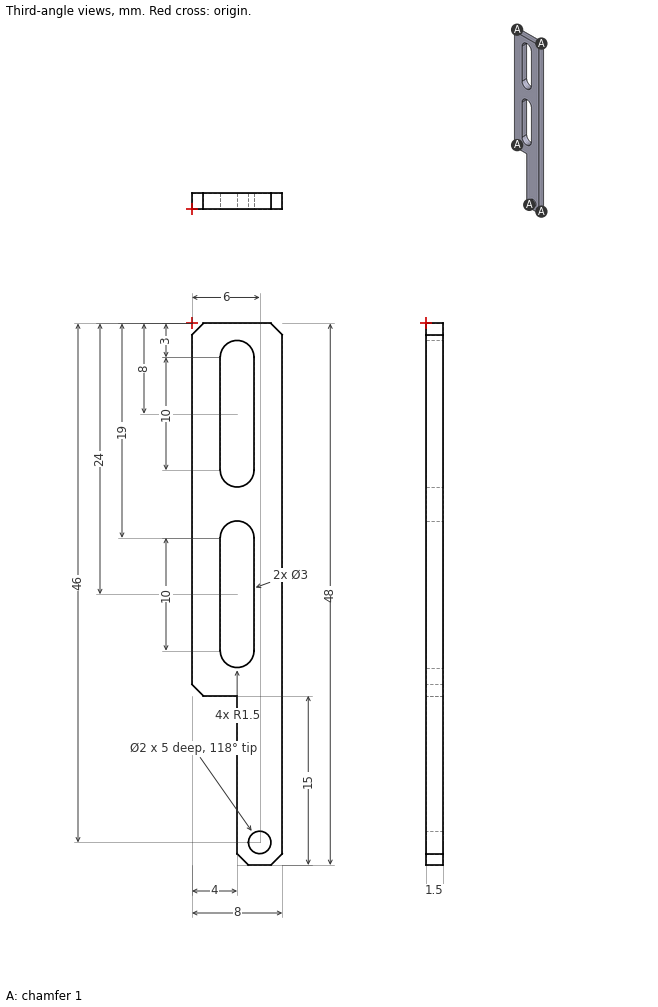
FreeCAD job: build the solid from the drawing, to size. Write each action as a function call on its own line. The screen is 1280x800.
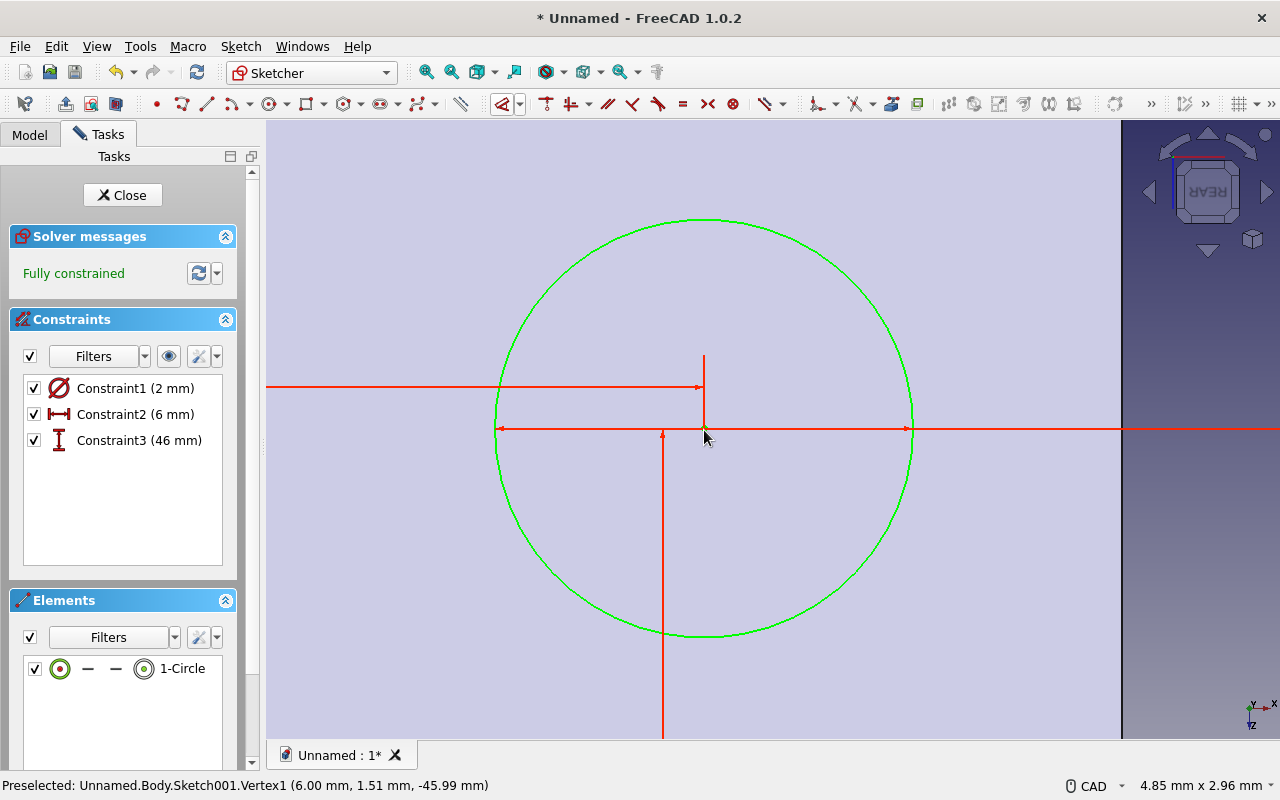
click(123, 195)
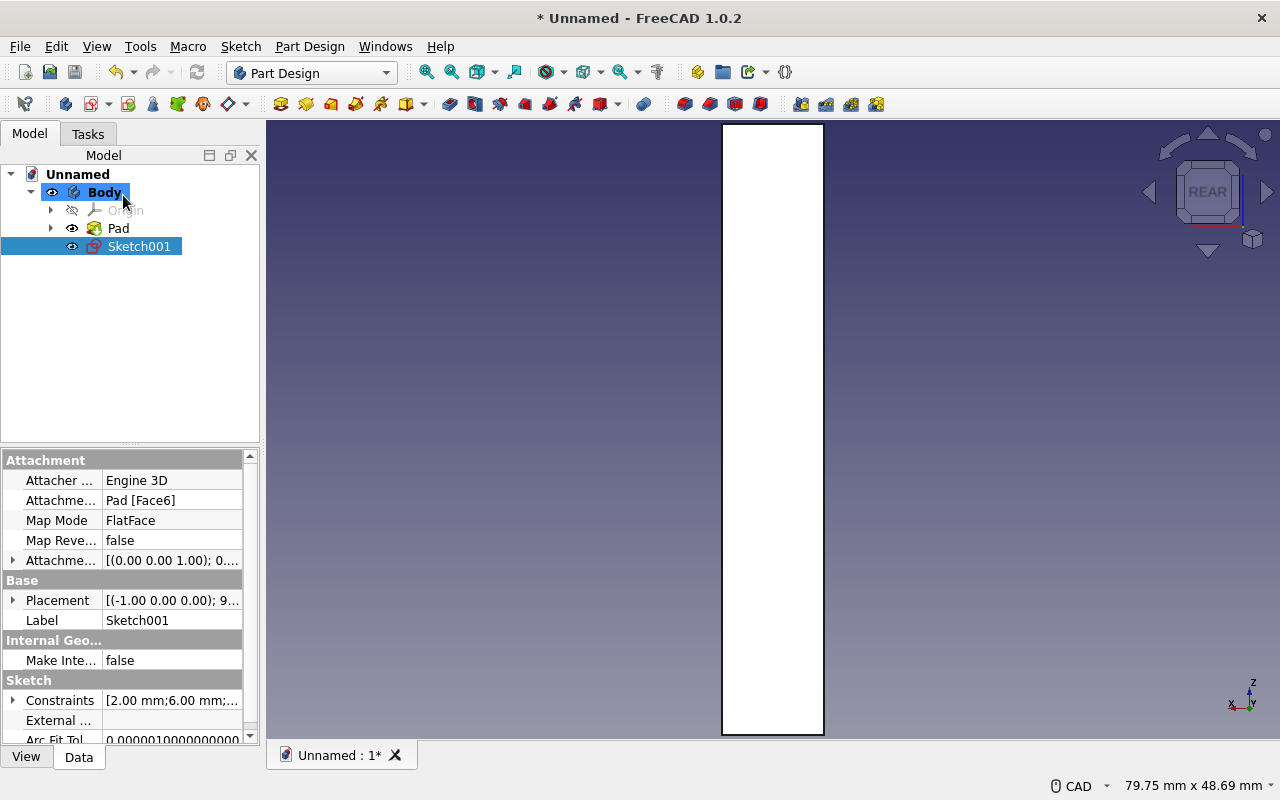
click(475, 104)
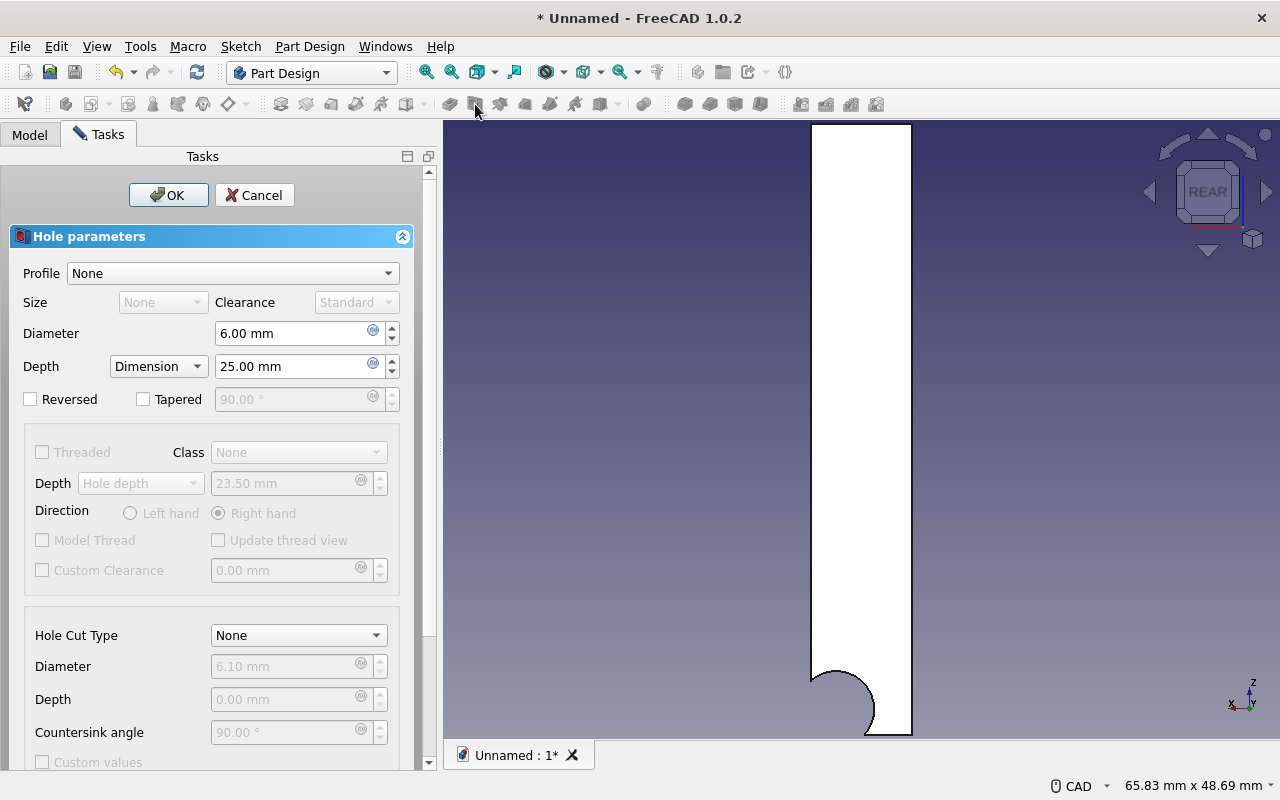
triple_click(300, 334)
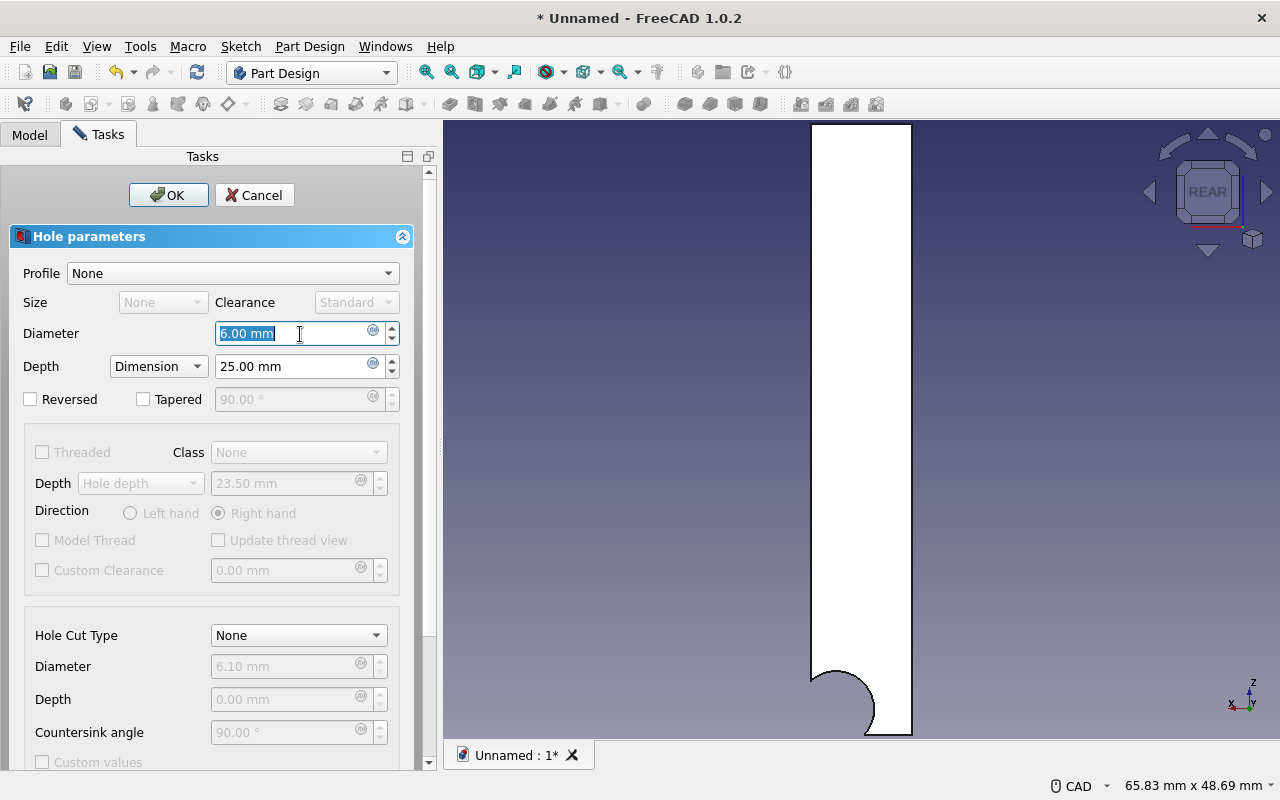
text(2)
key(Tab)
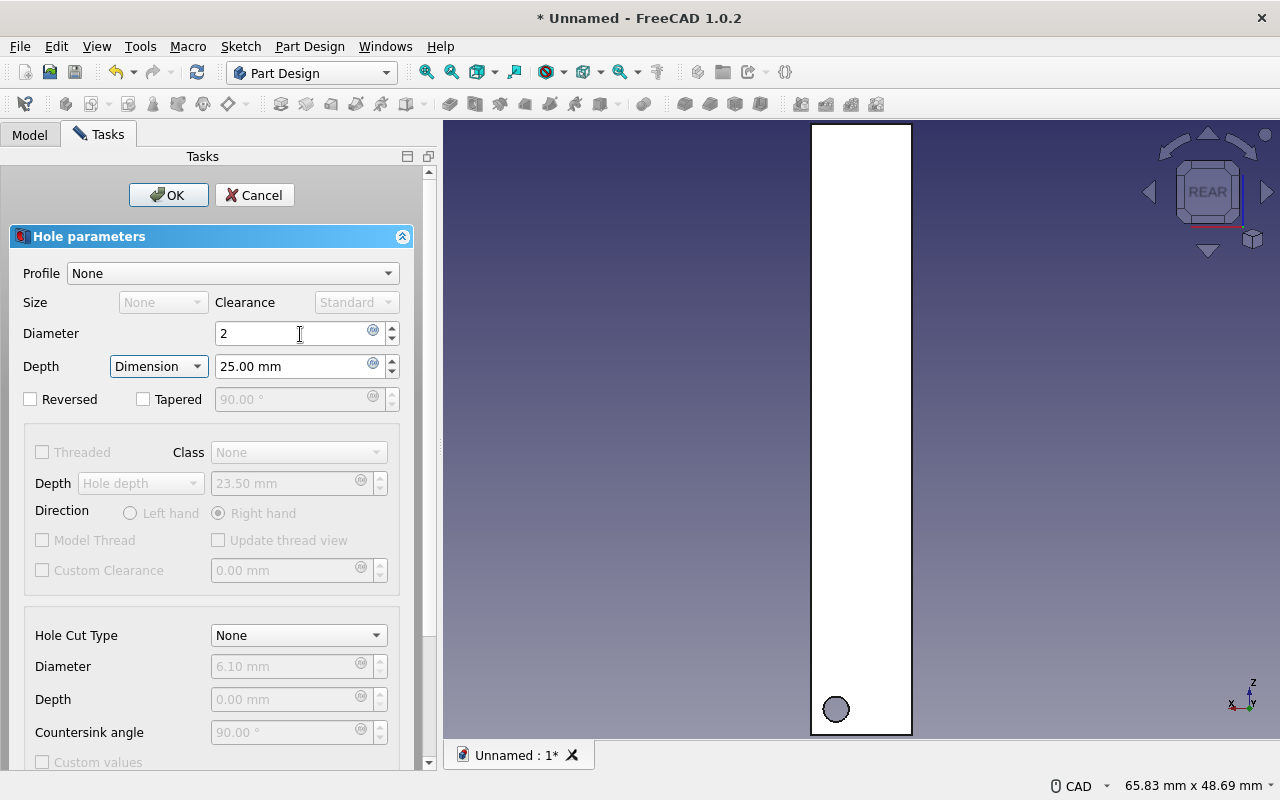
triple_click(300, 366)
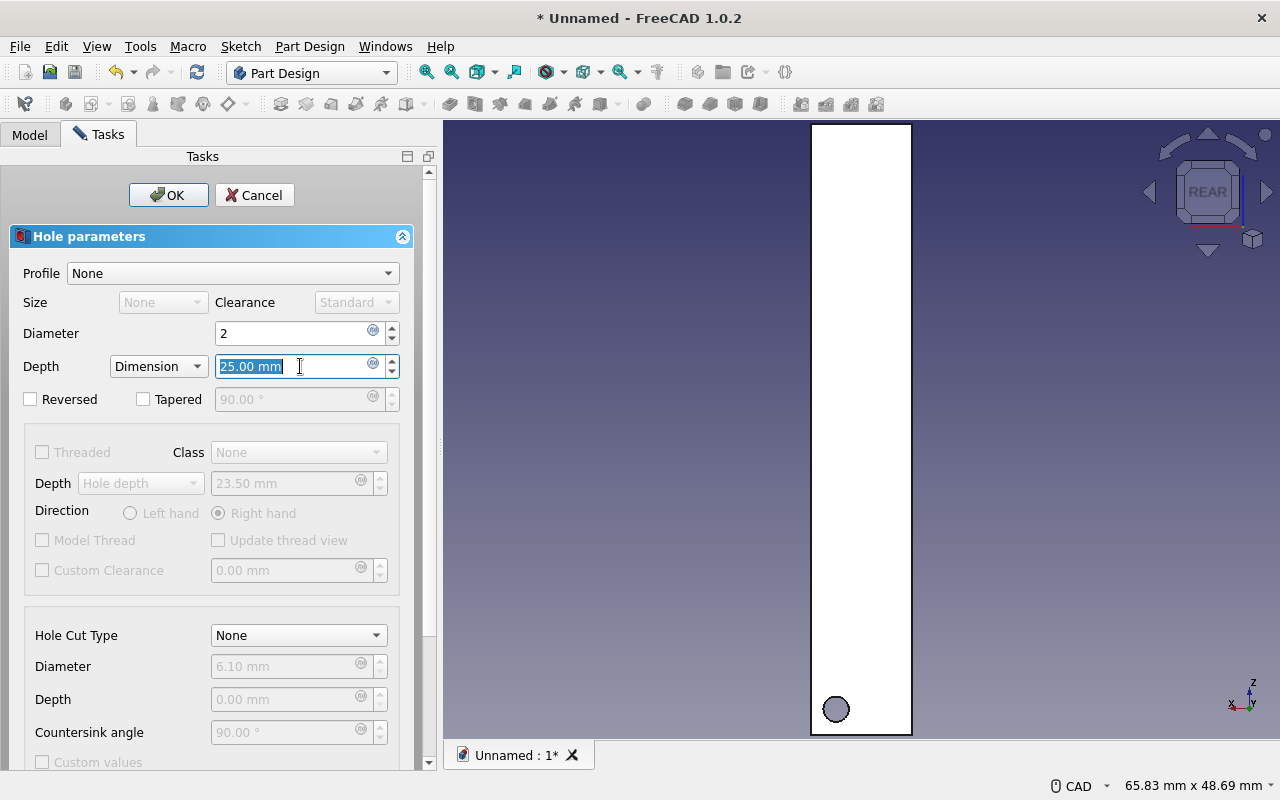
text(5)
key(Tab)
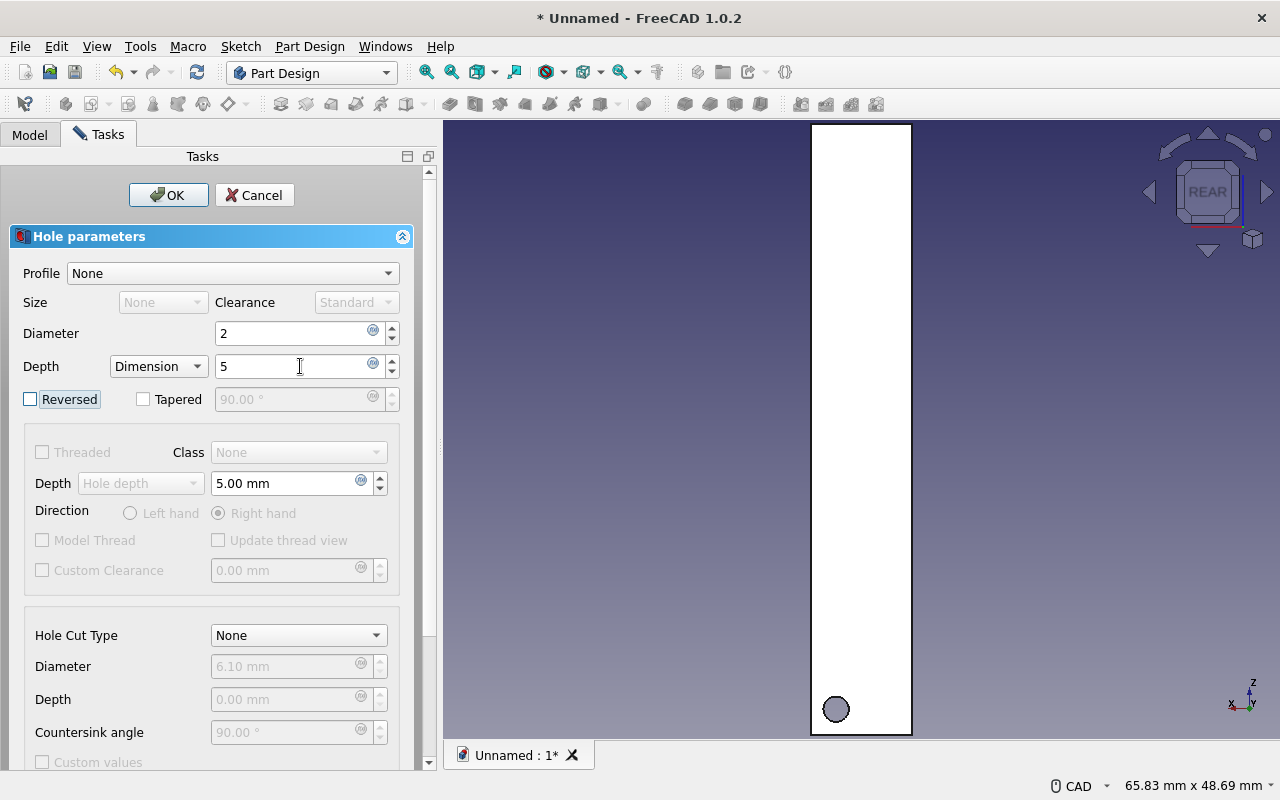
click(169, 195)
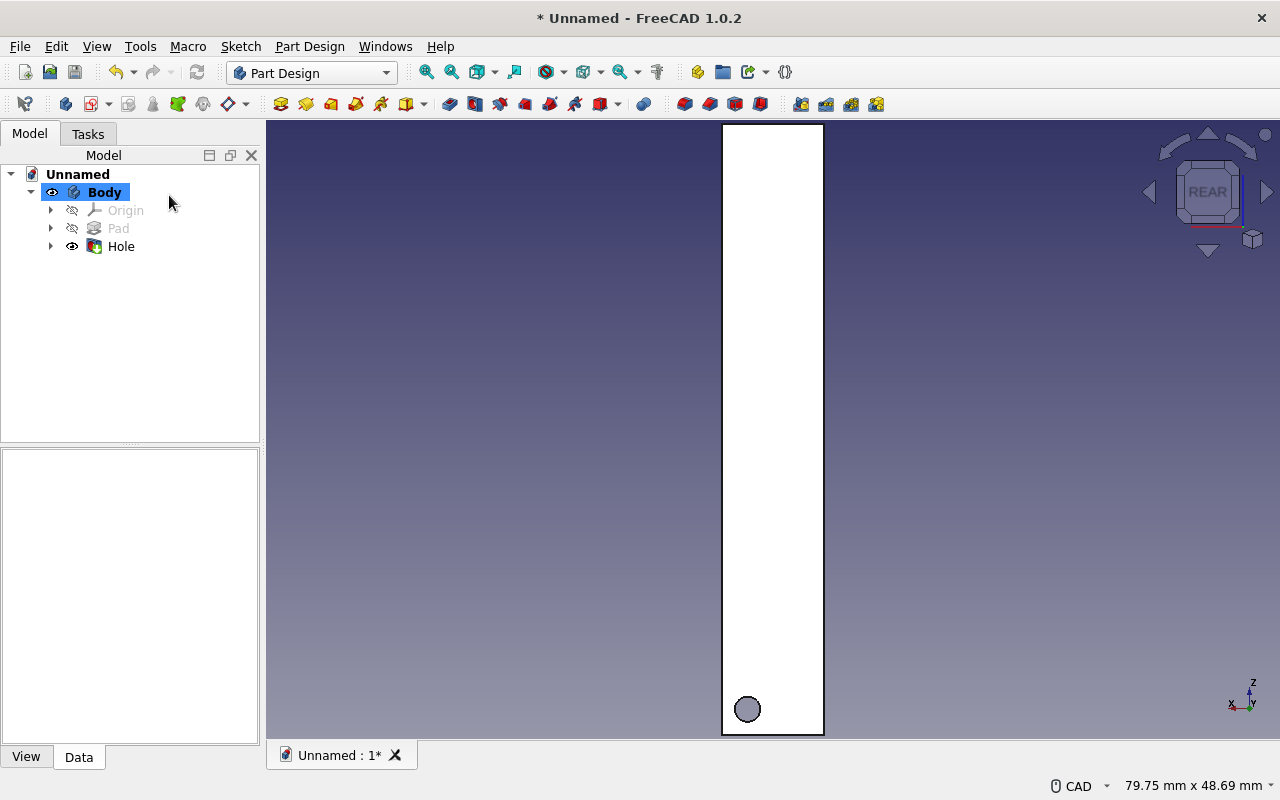
click(773, 254)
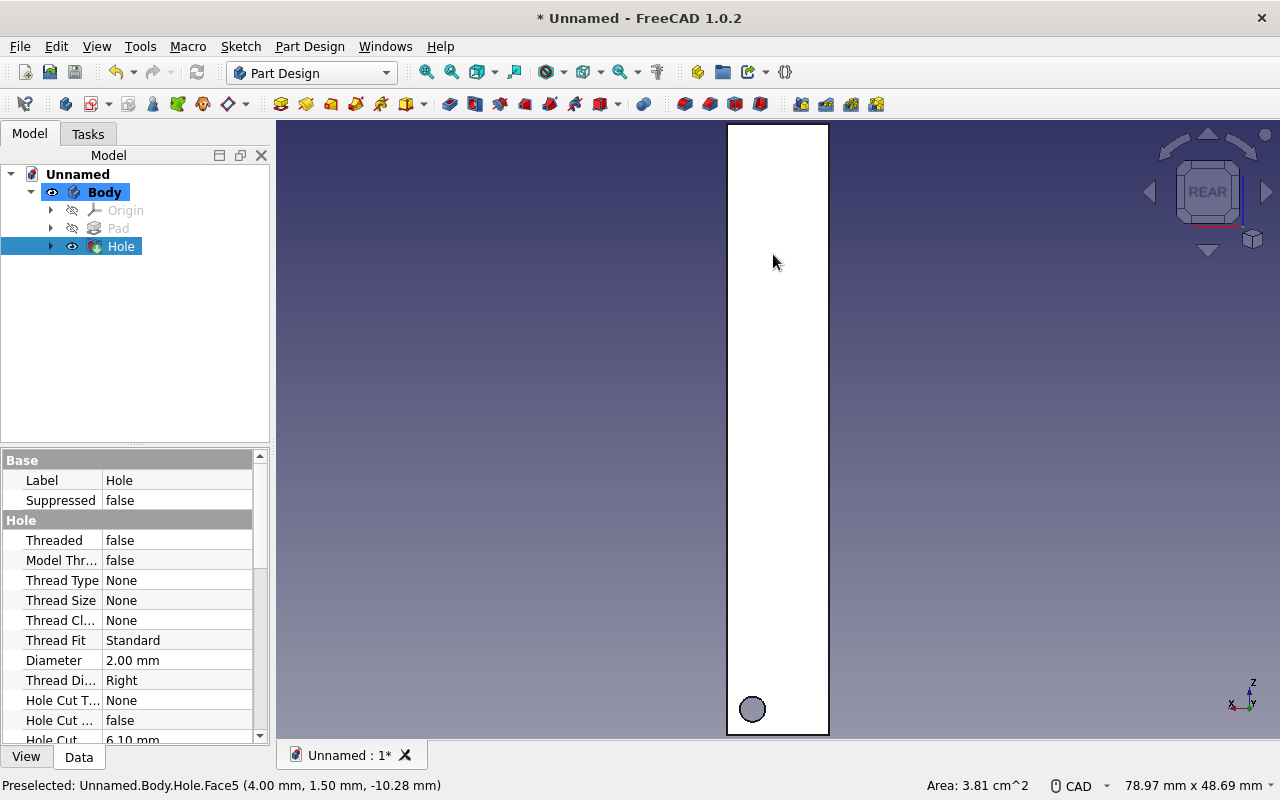
click(90, 104)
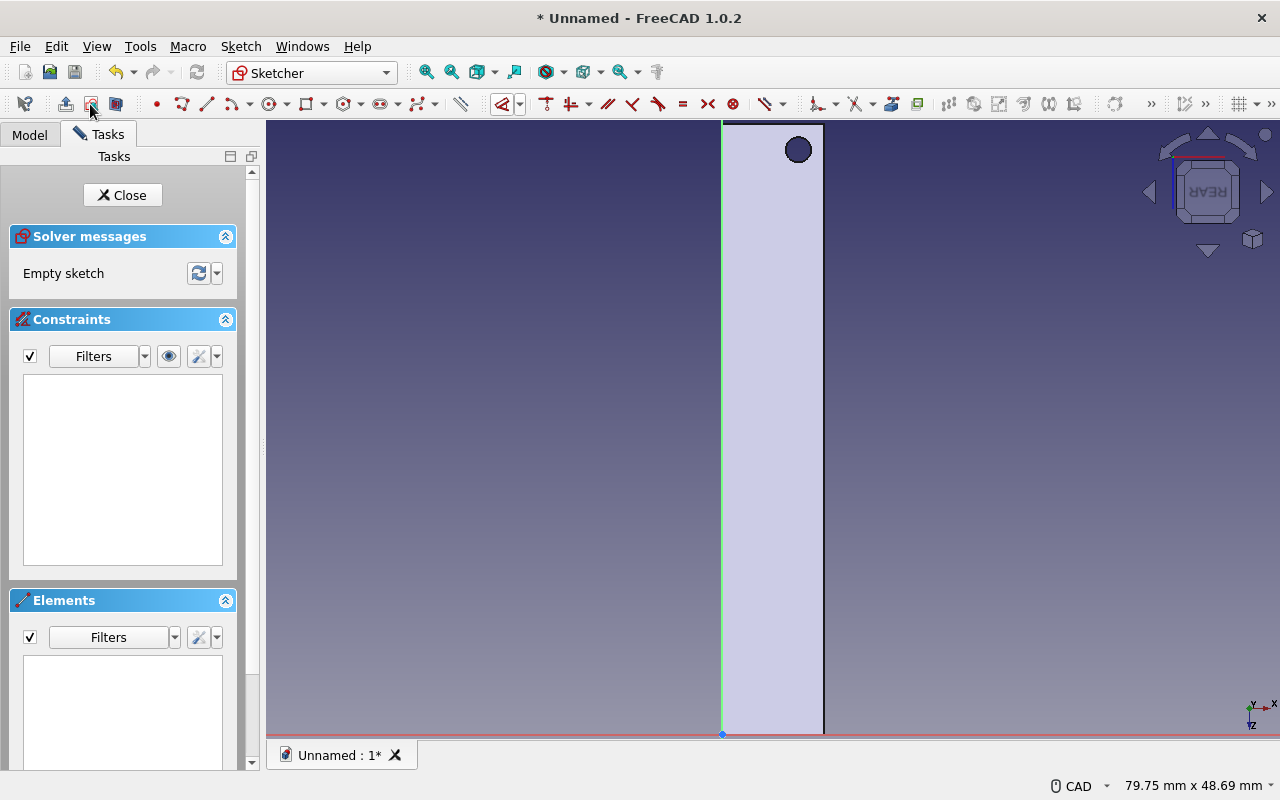
scroll(704, 430, down, 5)